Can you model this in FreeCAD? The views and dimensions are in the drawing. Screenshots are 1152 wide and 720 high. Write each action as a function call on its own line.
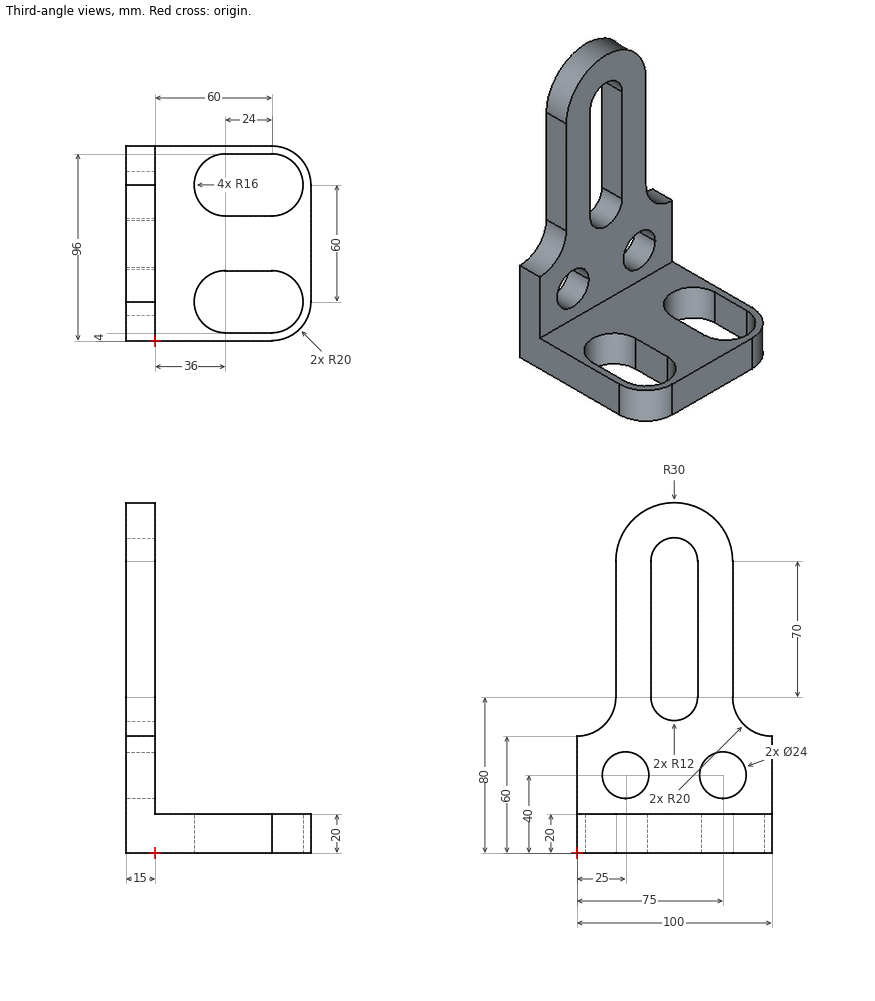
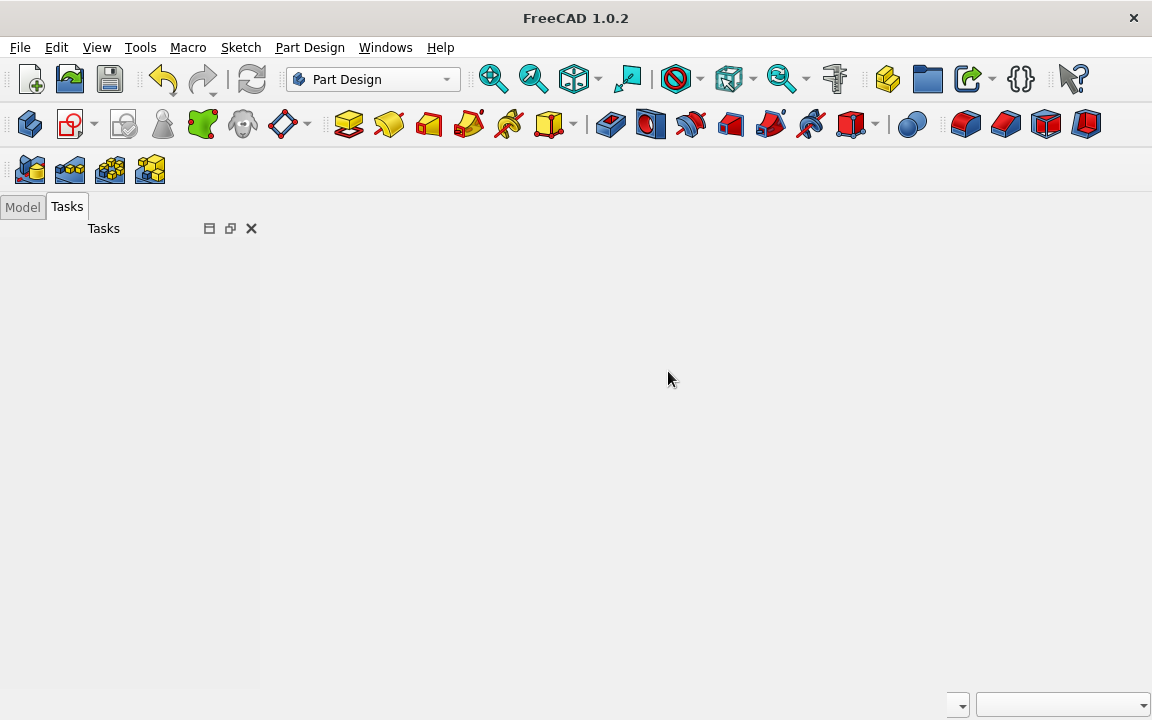
click(30, 80)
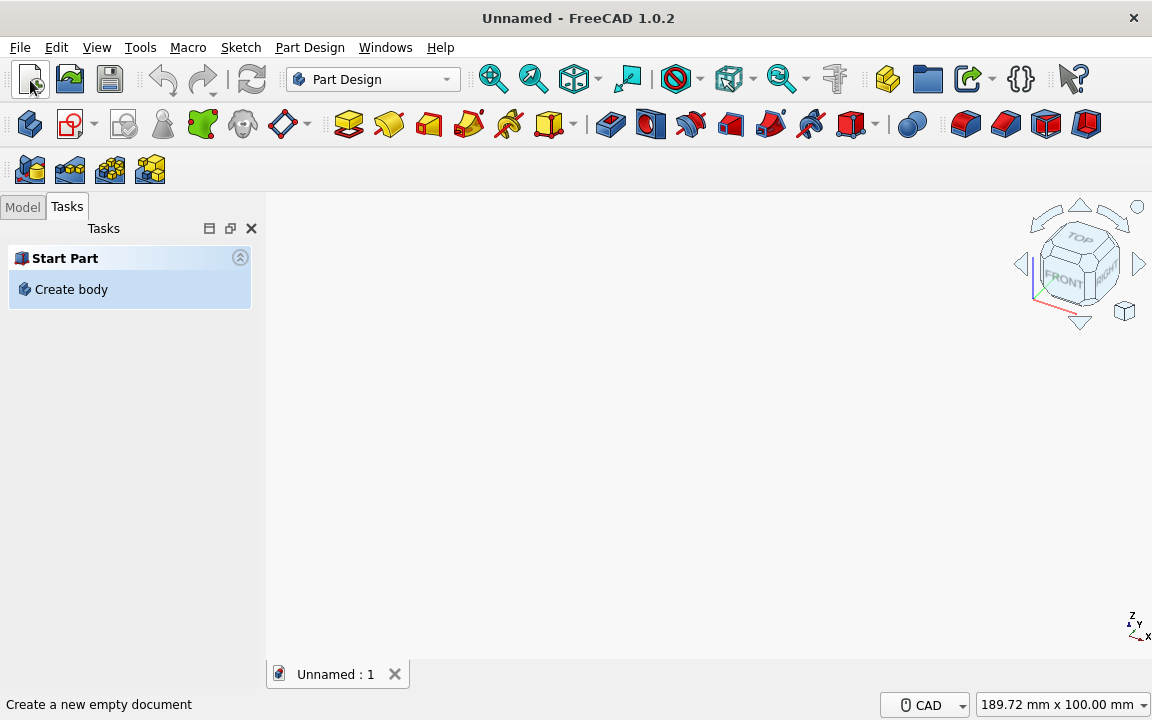
click(70, 124)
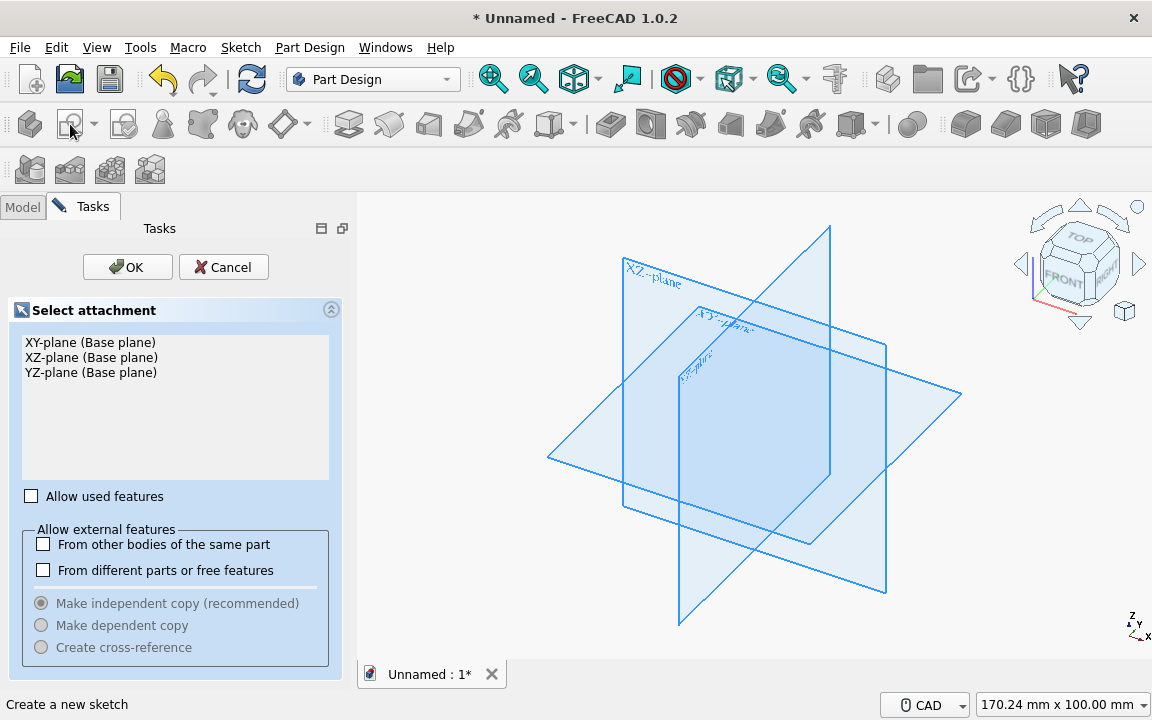
click(82, 342)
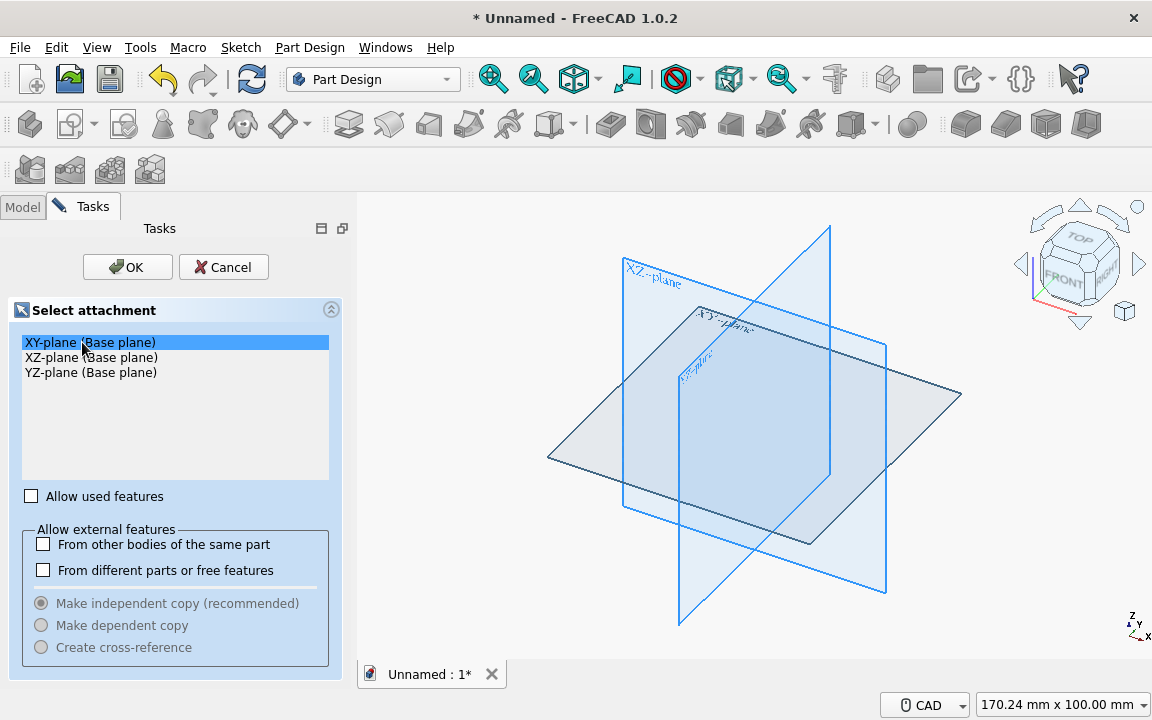
click(128, 267)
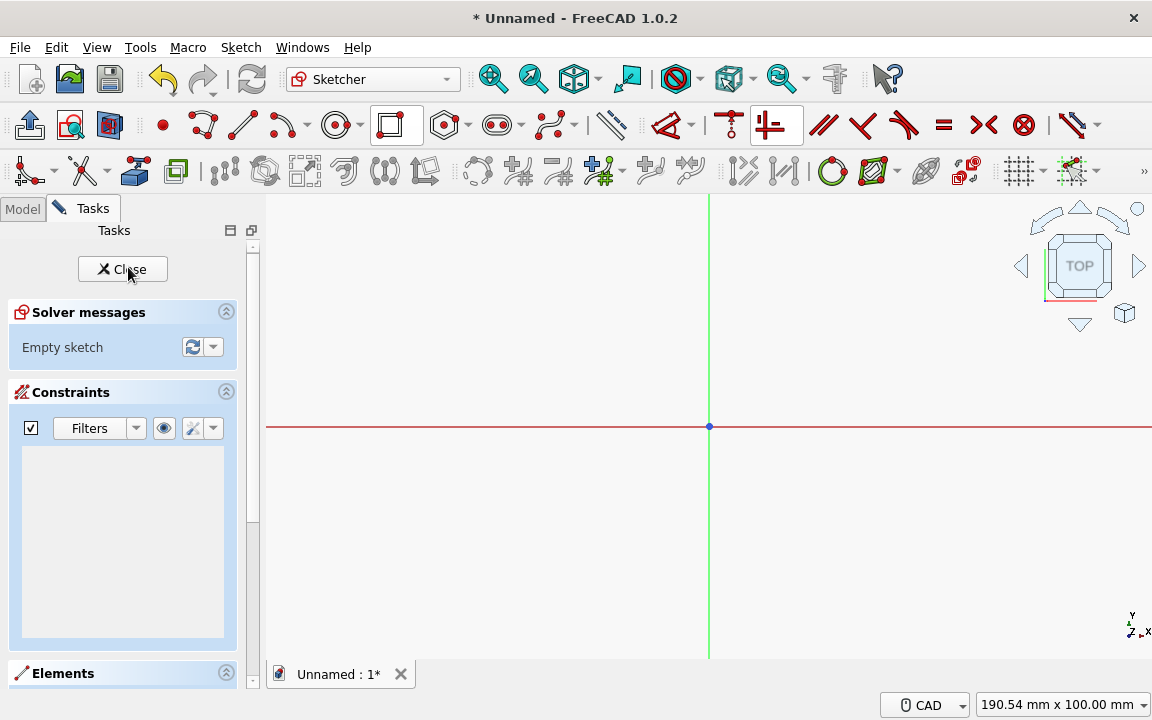
scroll(331, 631, down, 3)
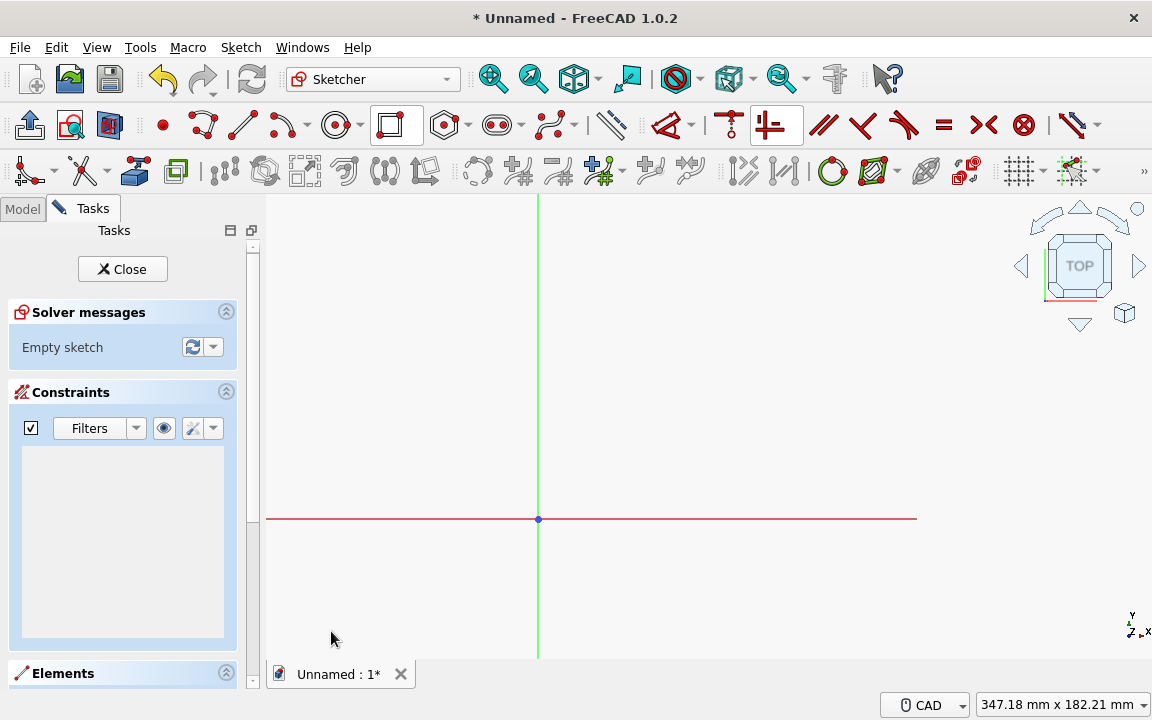
click(244, 126)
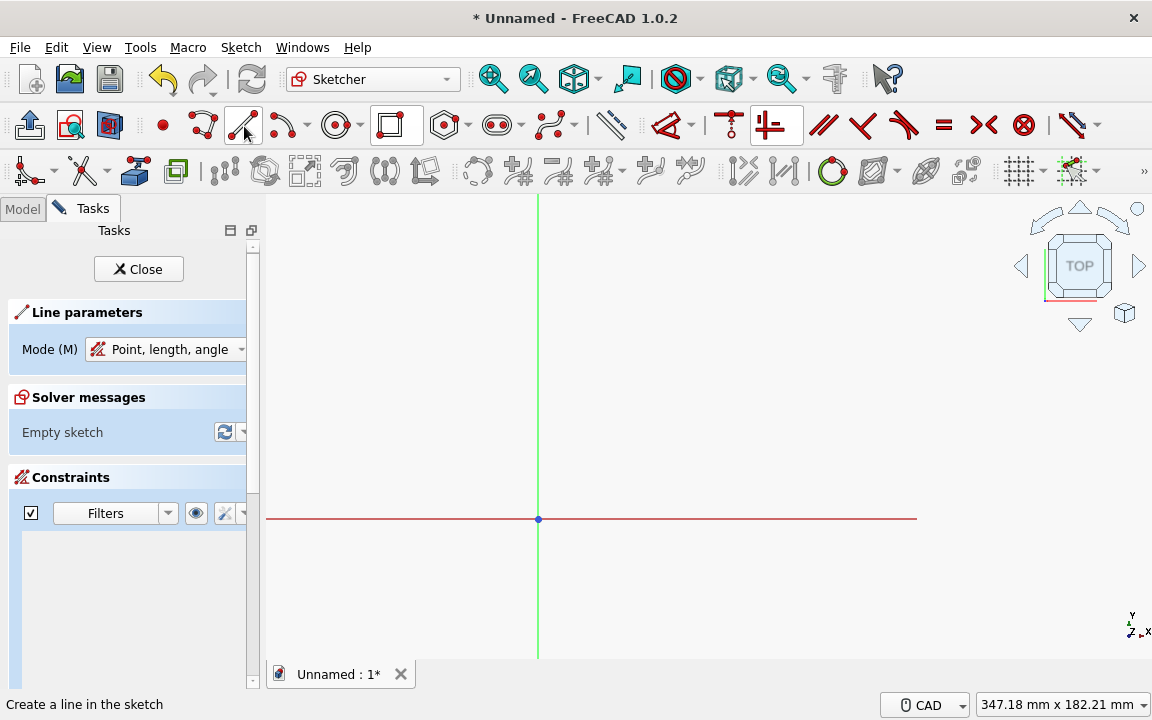
click(743, 468)
click(743, 315)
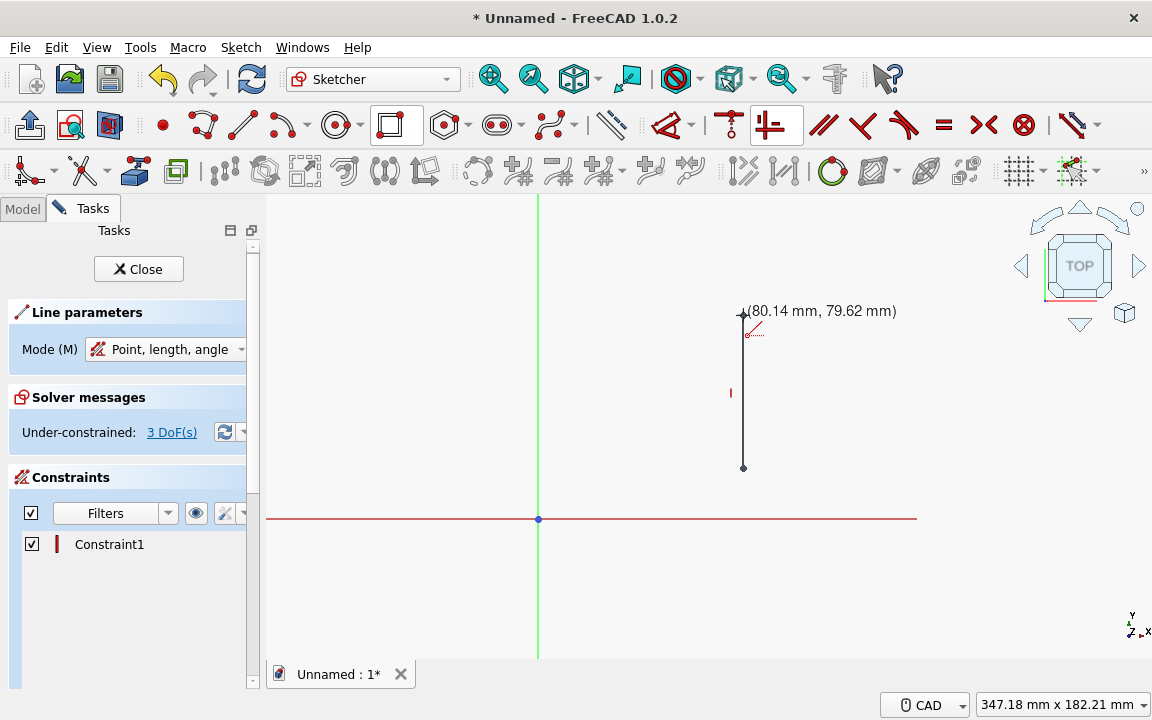
click(204, 126)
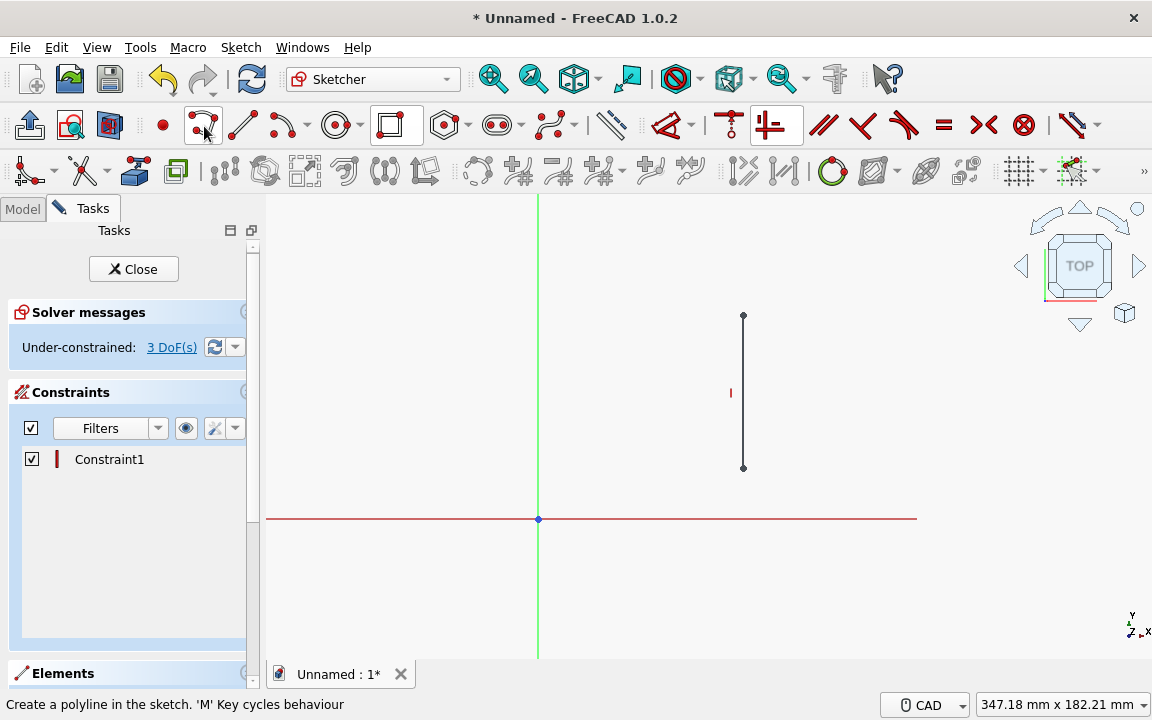
click(692, 264)
click(538, 264)
click(538, 519)
click(692, 510)
right_click(692, 510)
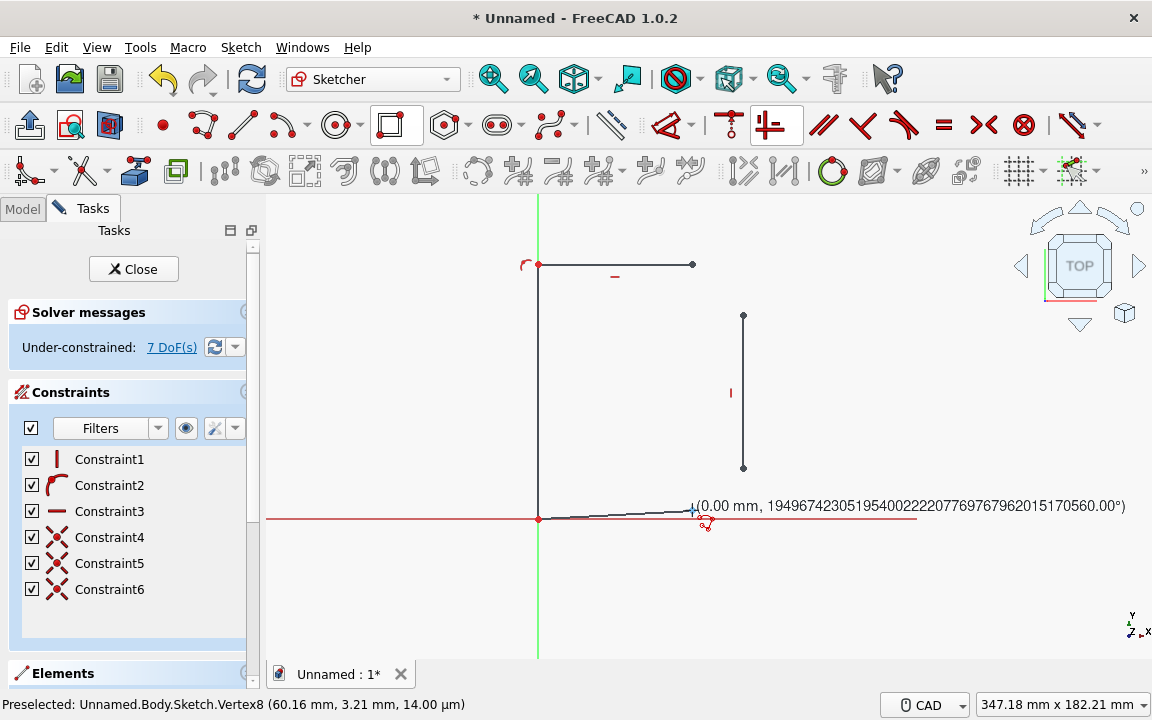
click(310, 126)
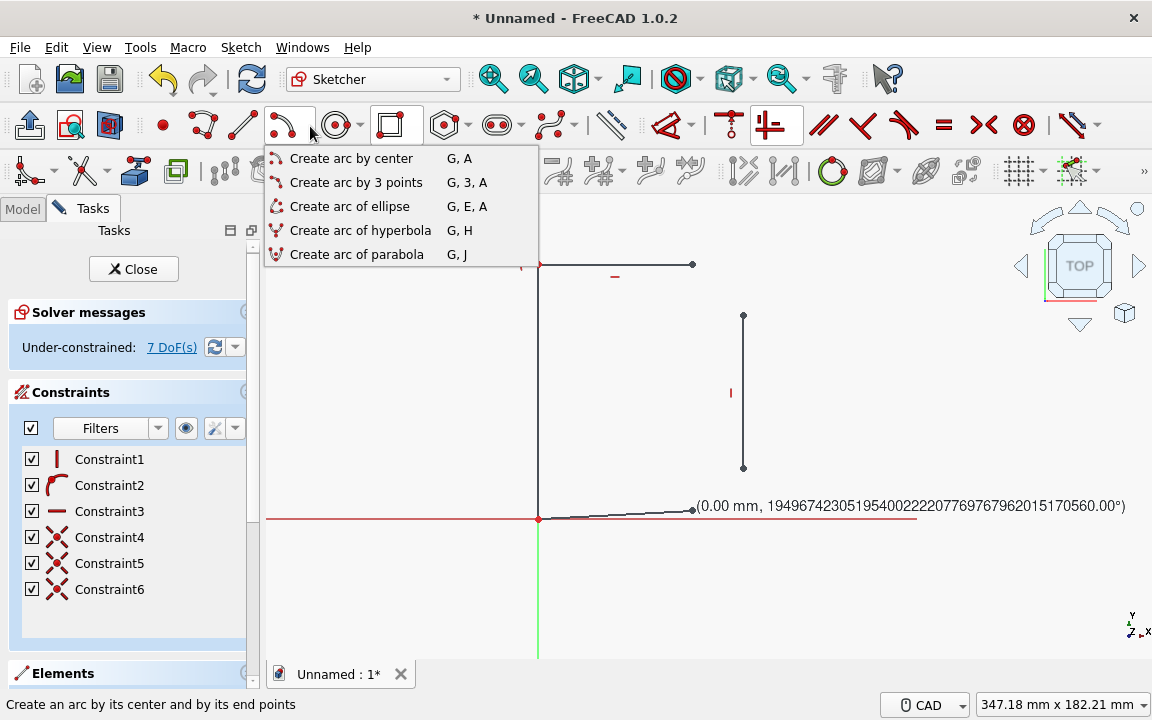
click(402, 182)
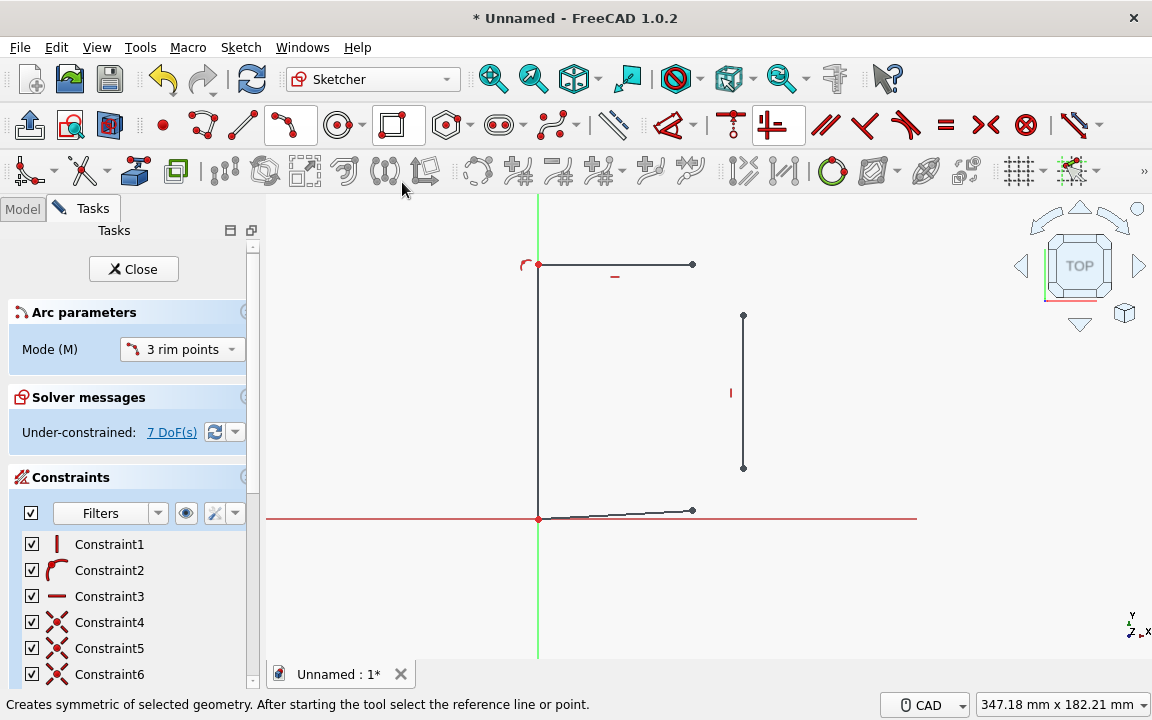
click(743, 316)
click(692, 265)
click(728, 279)